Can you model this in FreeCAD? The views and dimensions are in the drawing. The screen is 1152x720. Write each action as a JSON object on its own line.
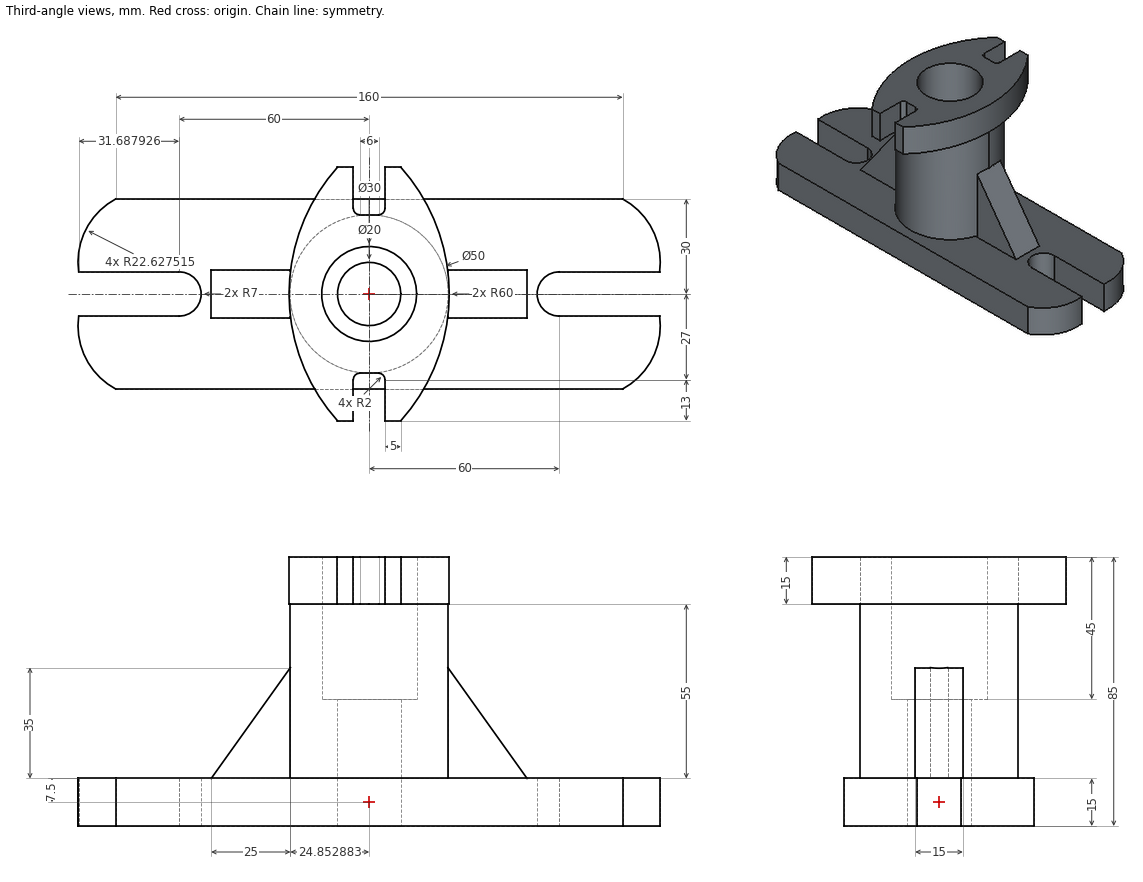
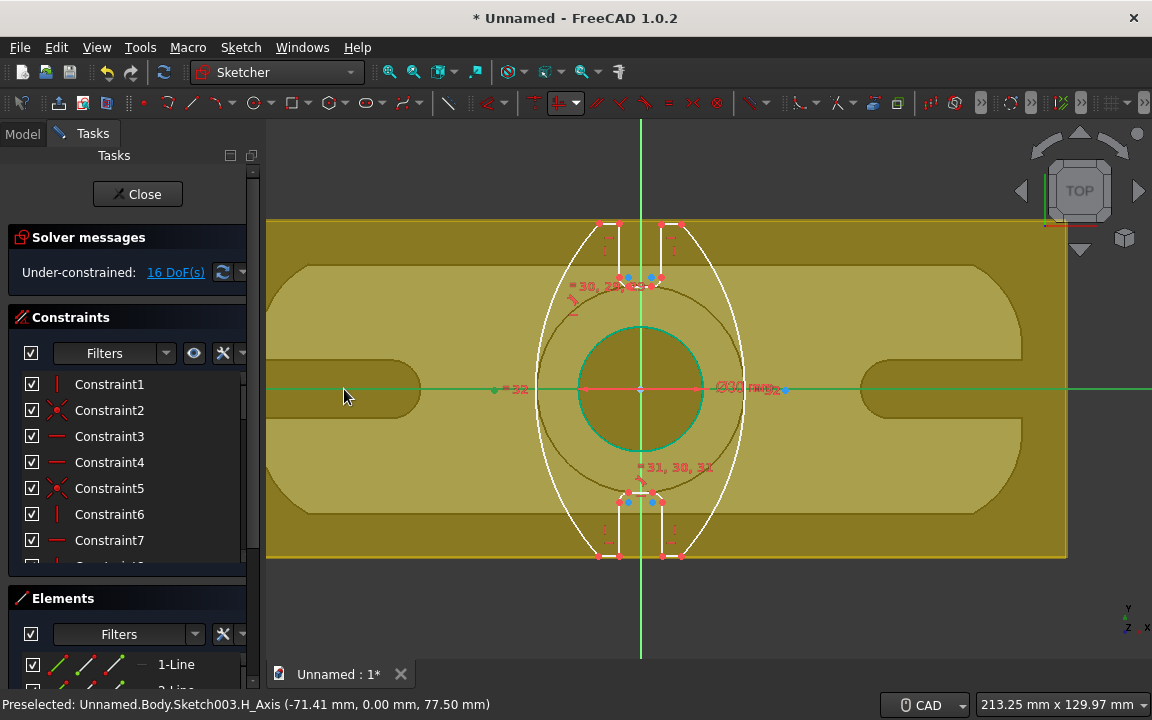
{"action": "left_click", "coordinate": [534, 104]}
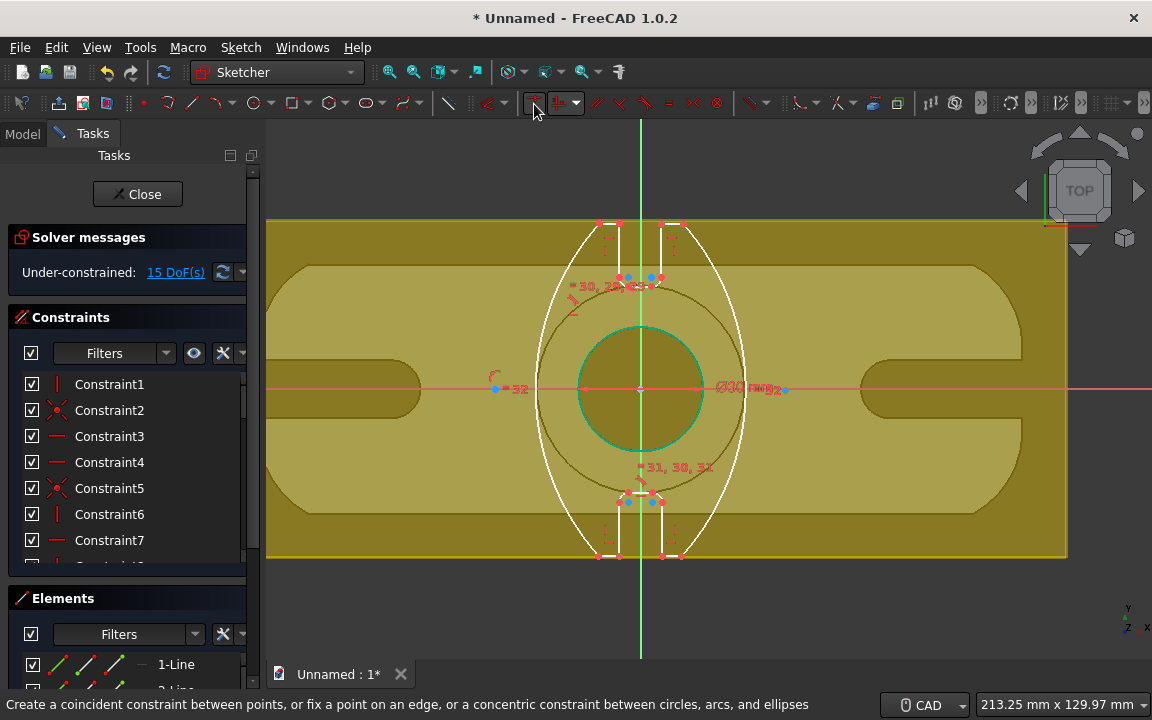
{"action": "left_click", "coordinate": [786, 390]}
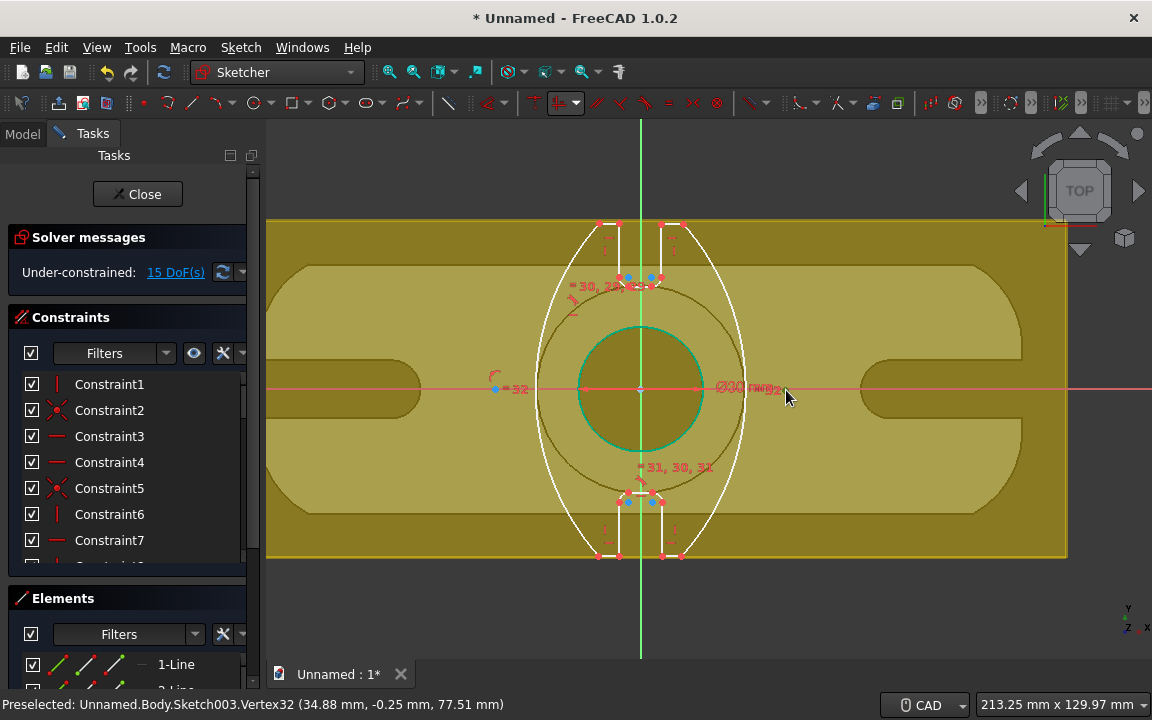
{"action": "left_click", "coordinate": [344, 389]}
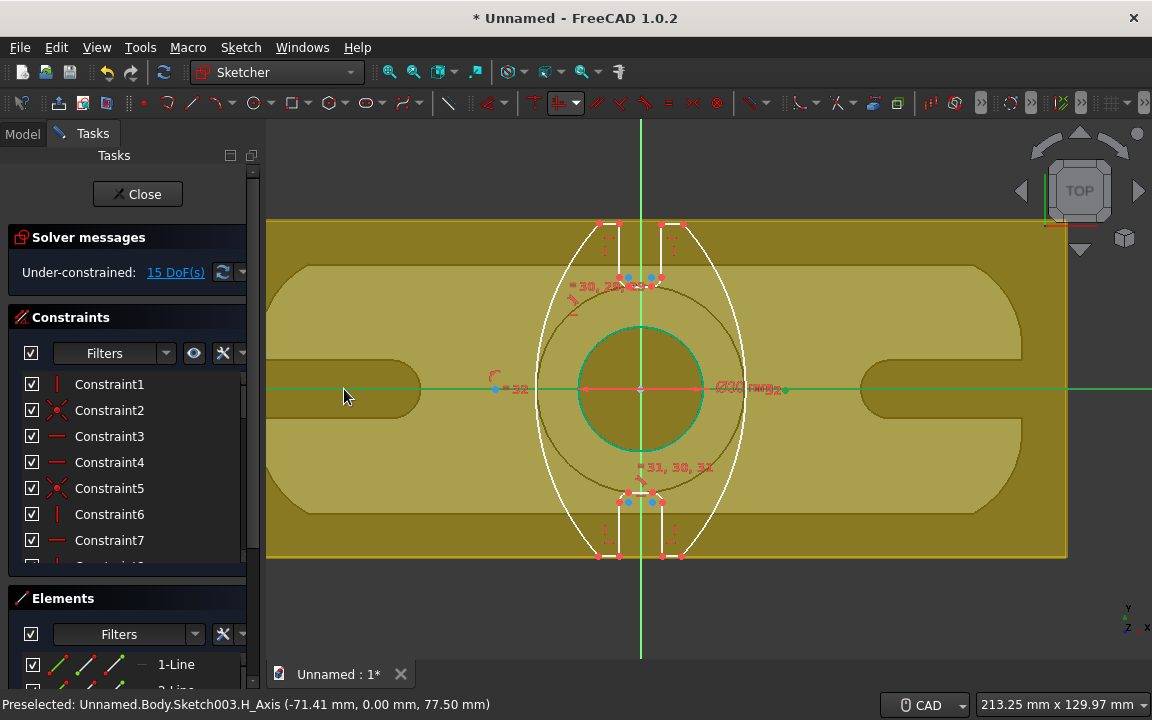
{"action": "left_click", "coordinate": [534, 104]}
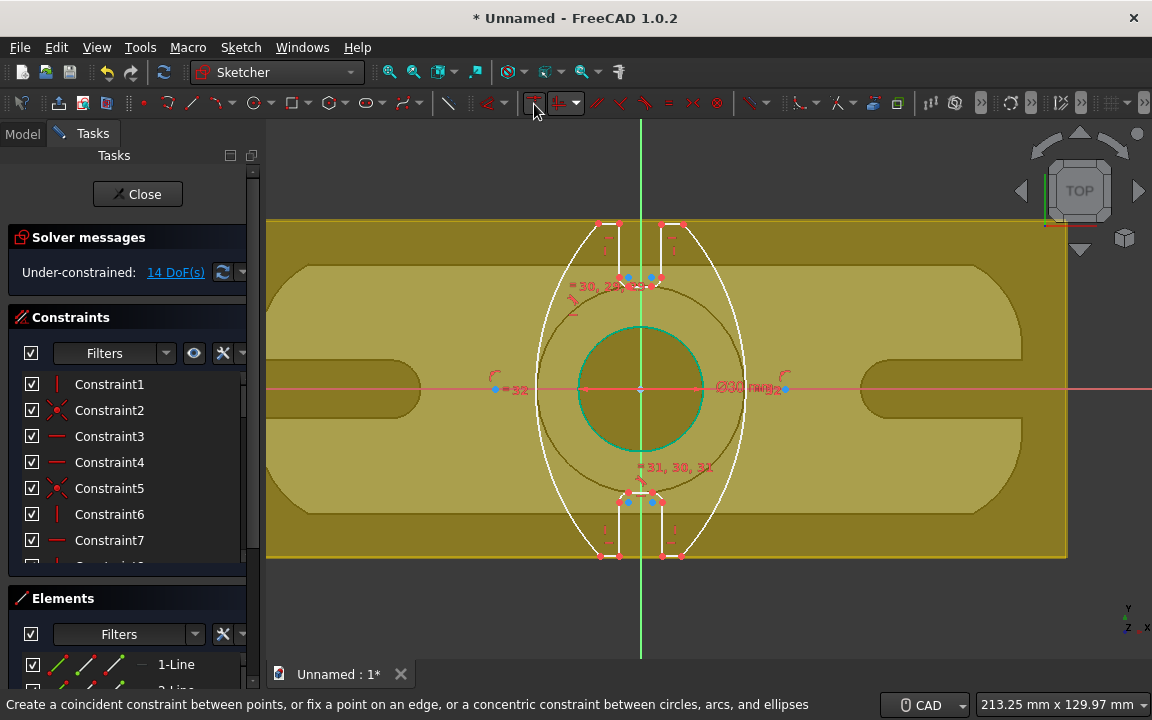
{"action": "scroll", "coordinate": [629, 277], "scroll_direction": "up", "scroll_amount": 2}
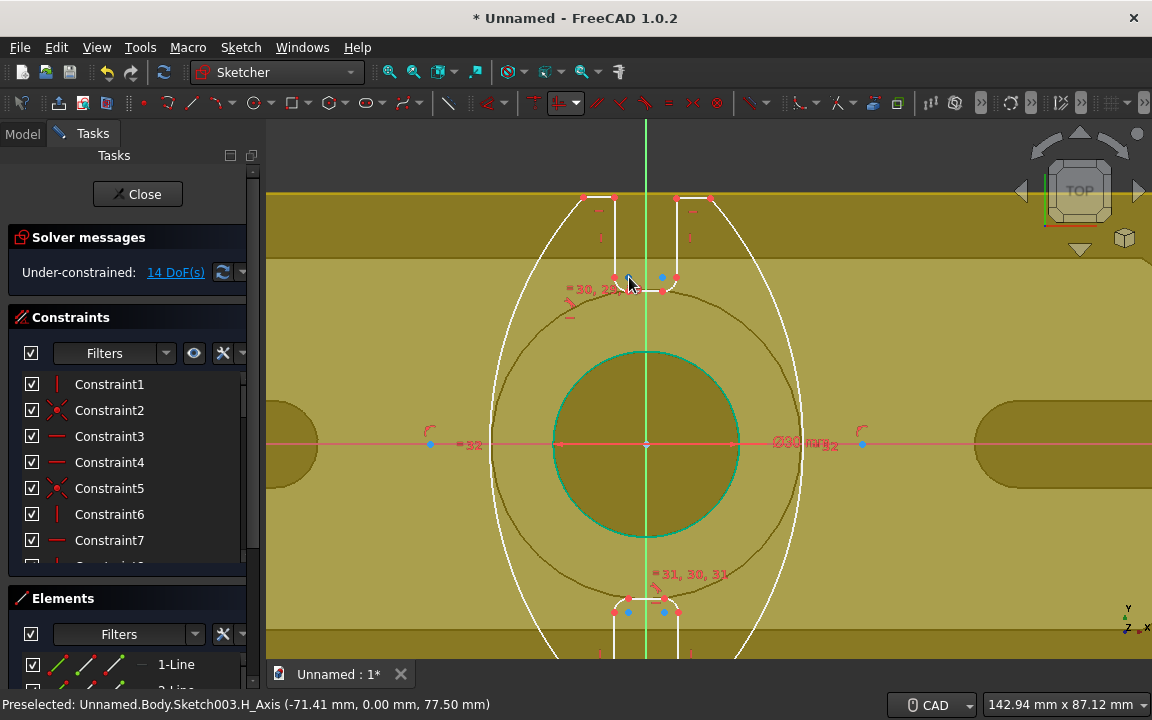
{"action": "left_click", "coordinate": [629, 277]}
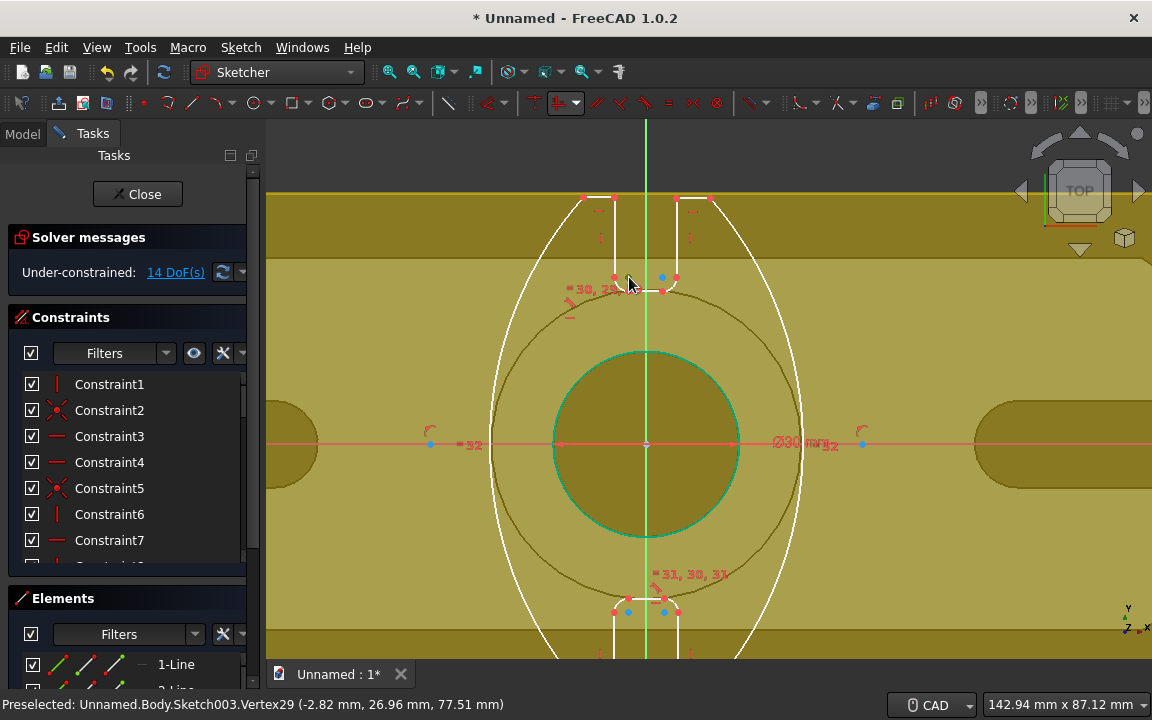
{"action": "left_click", "coordinate": [628, 613]}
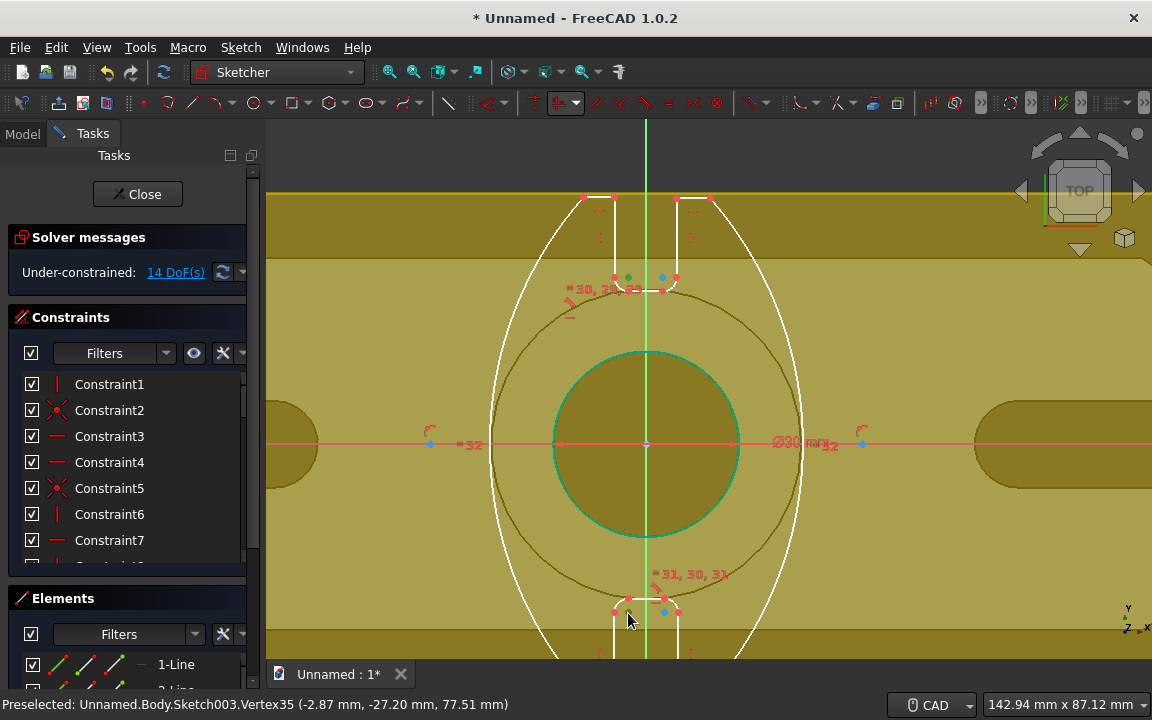
{"action": "left_click", "coordinate": [343, 444]}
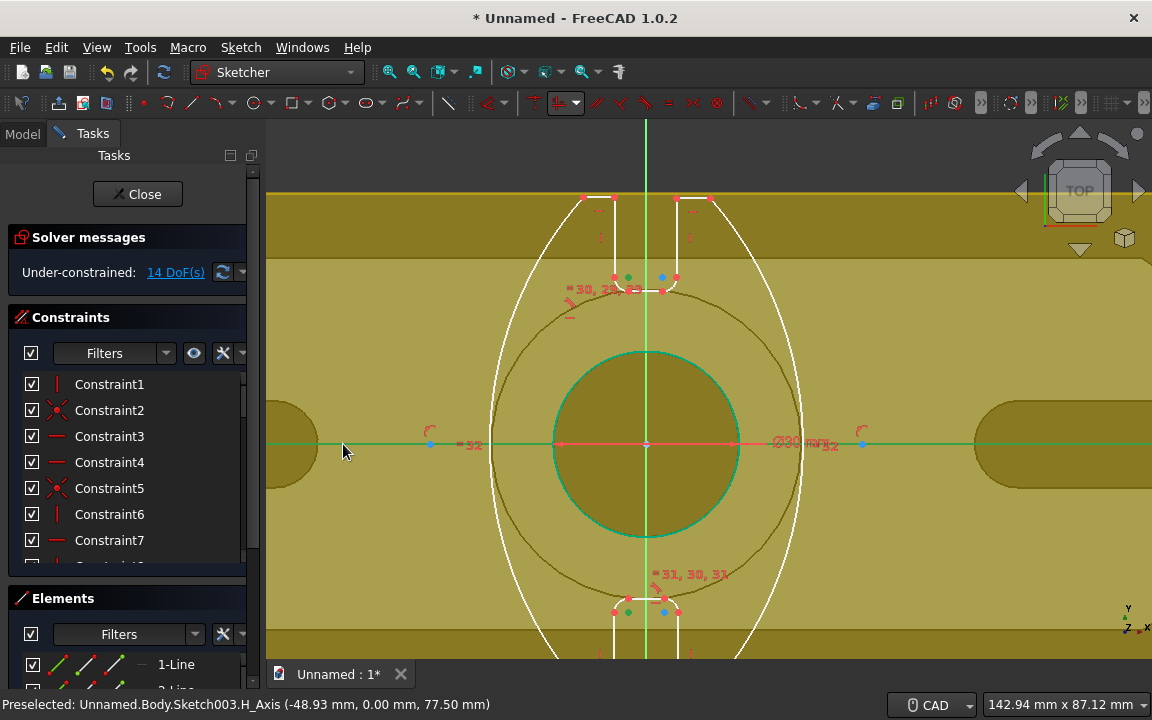
{"action": "key", "text": "s"}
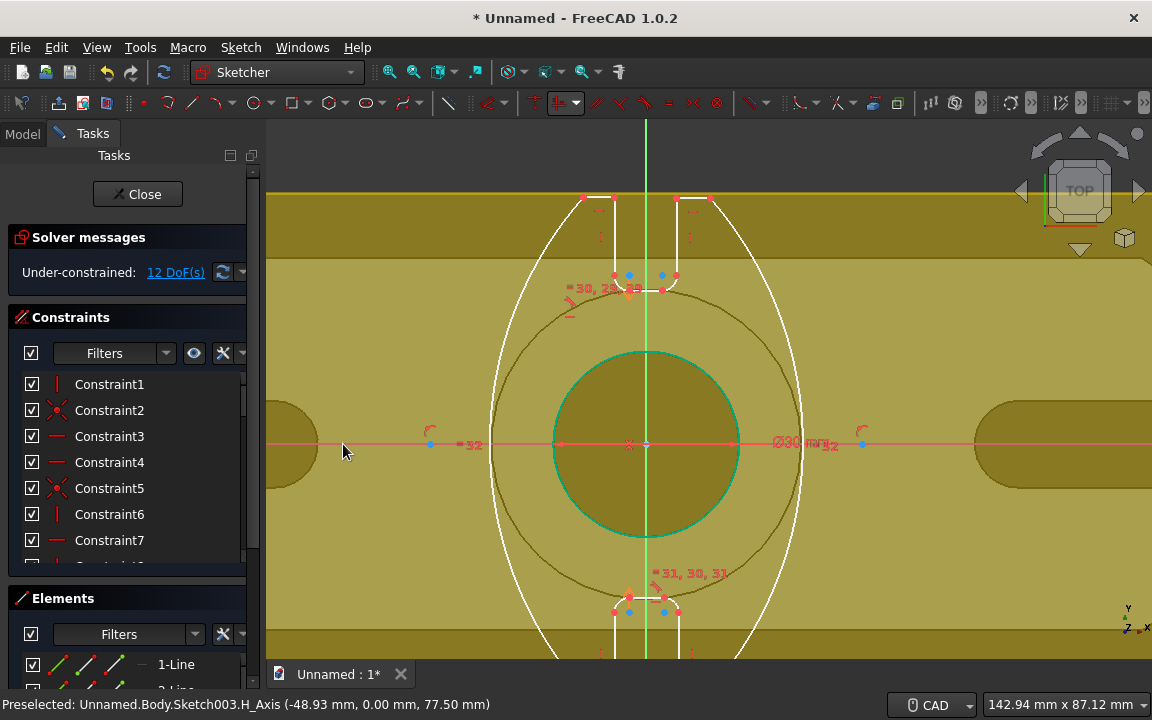
{"action": "scroll", "coordinate": [629, 277], "scroll_direction": "down", "scroll_amount": 2}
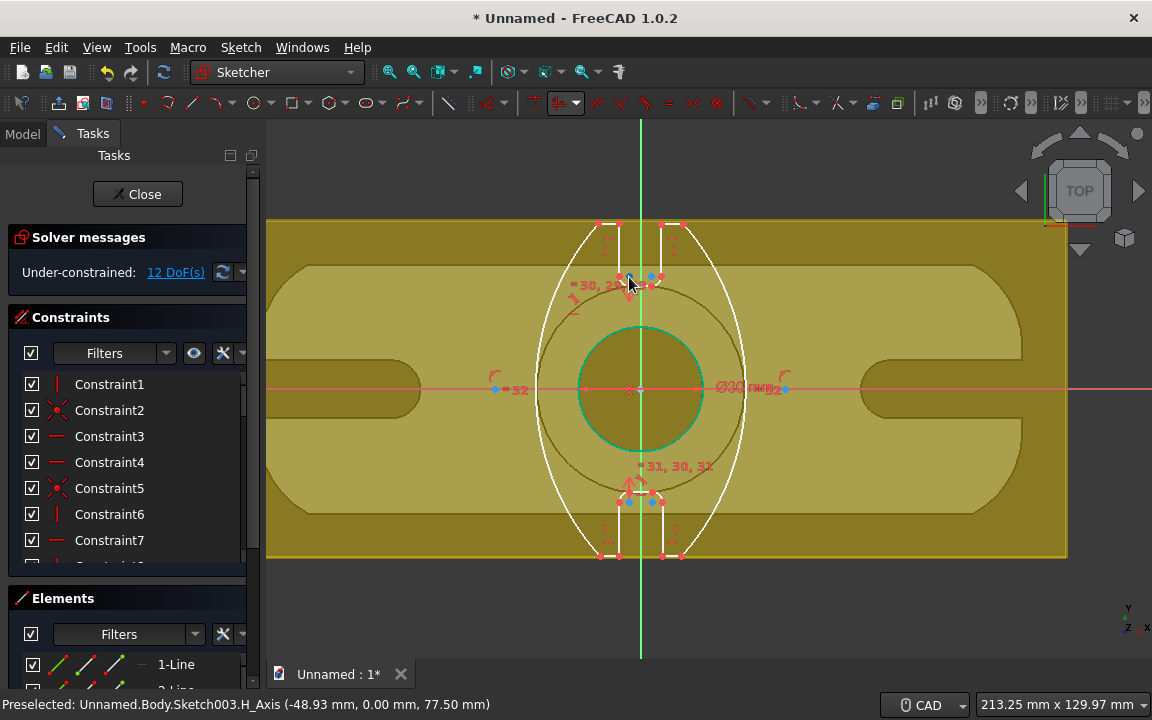
{"action": "left_click", "coordinate": [663, 556]}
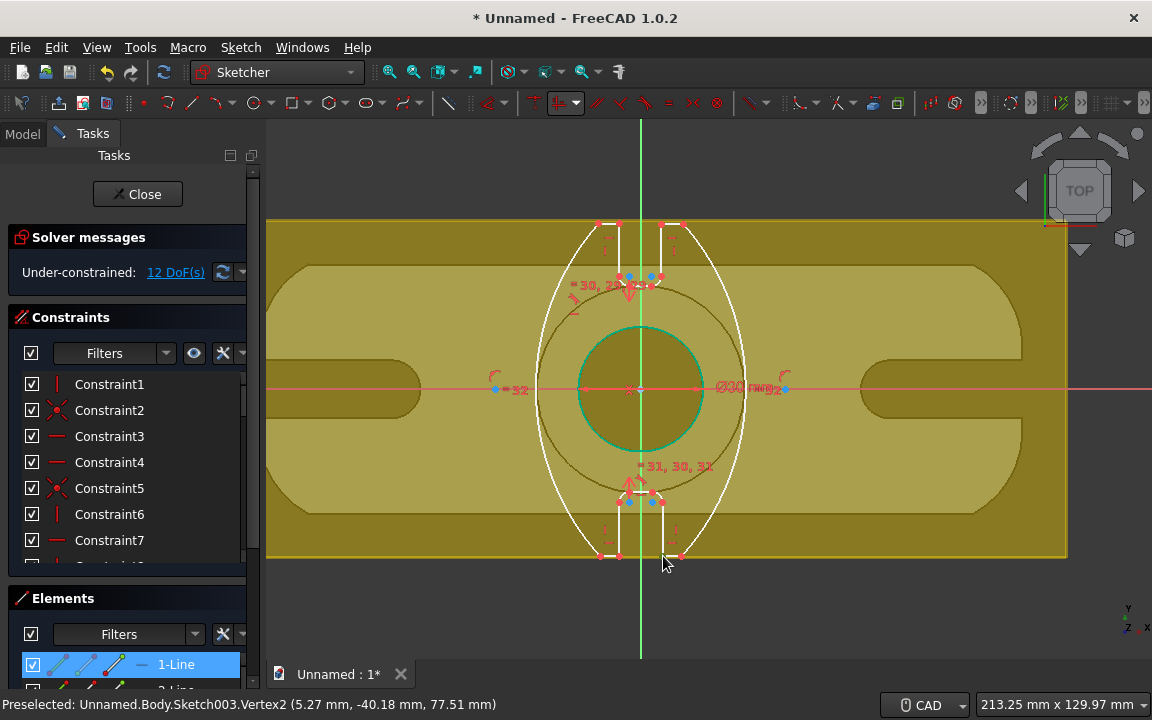
{"action": "left_click", "coordinate": [661, 224]}